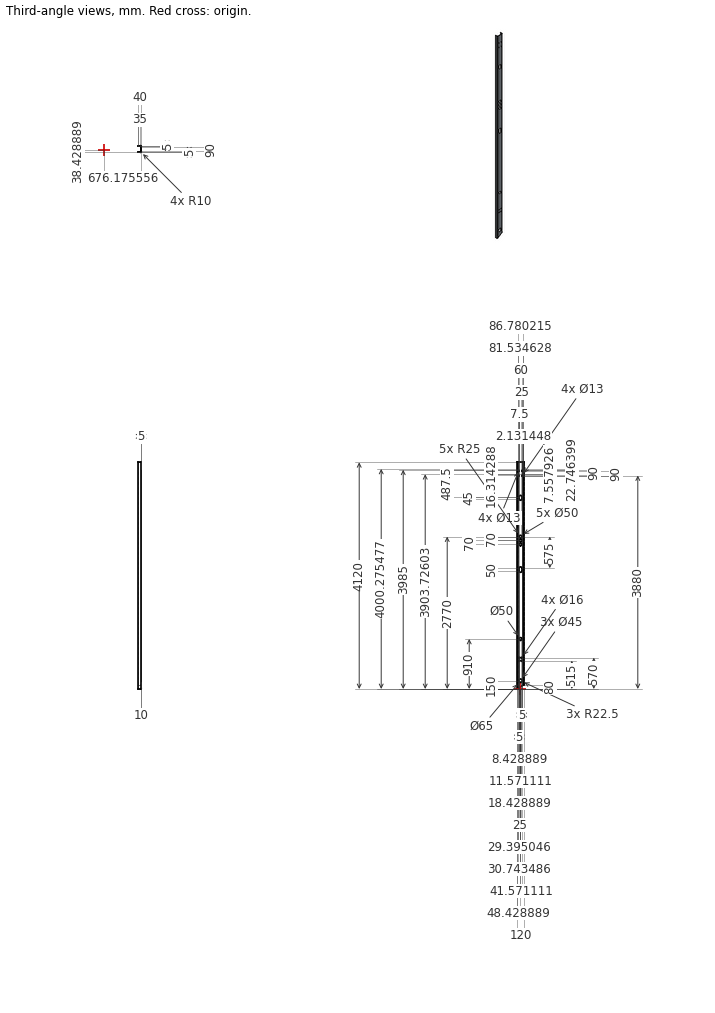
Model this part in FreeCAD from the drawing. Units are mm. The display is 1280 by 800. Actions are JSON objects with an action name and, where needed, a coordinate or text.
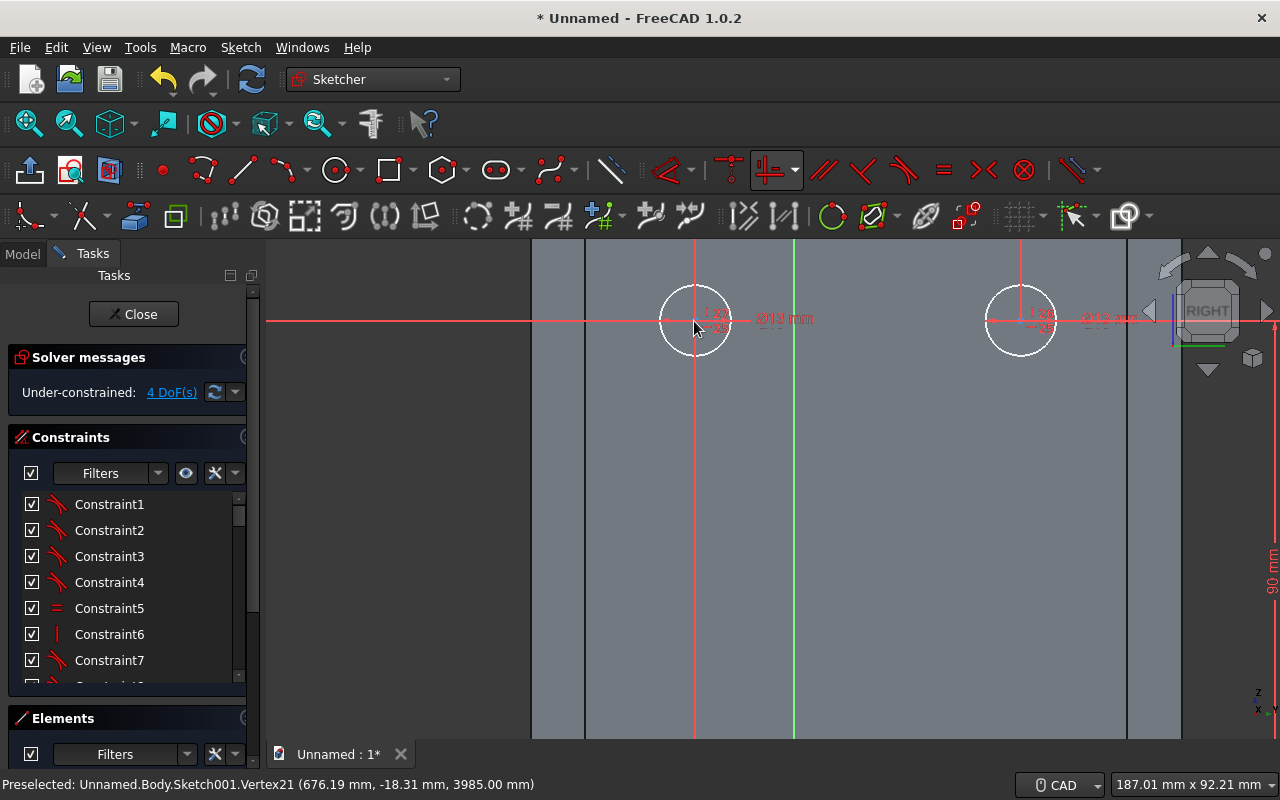
{"action": "scroll", "coordinate": [704, 489], "scroll_direction": "down", "scroll_amount": 15}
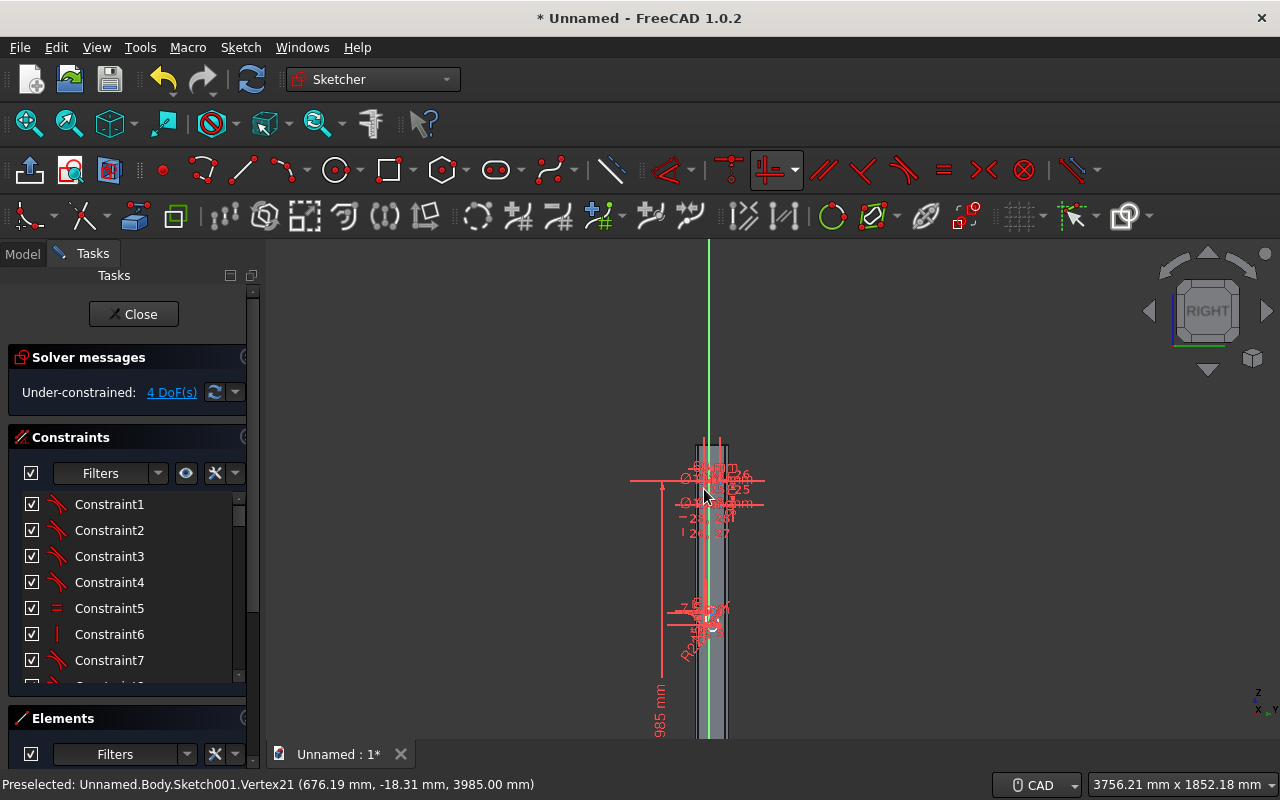
{"action": "scroll", "coordinate": [701, 267], "scroll_direction": "down", "scroll_amount": 6}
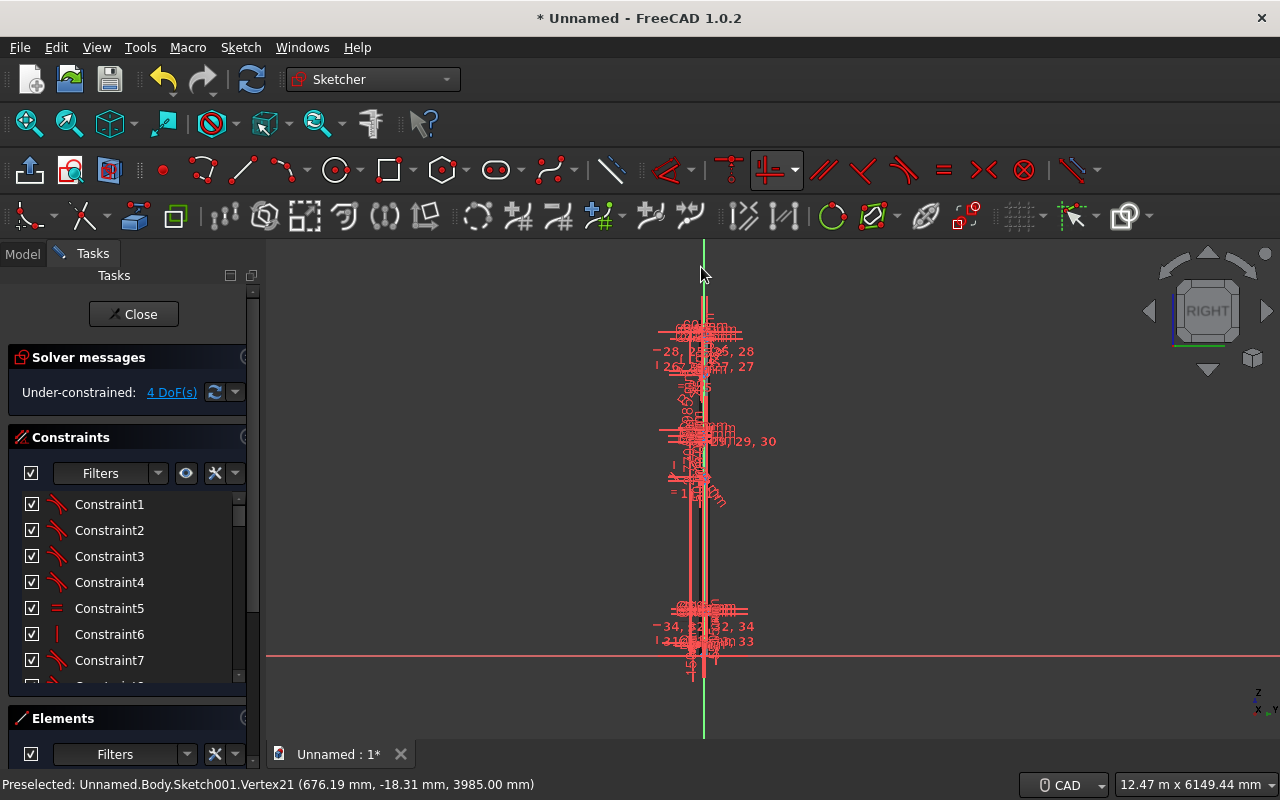
{"action": "scroll", "coordinate": [707, 477], "scroll_direction": "up", "scroll_amount": 9}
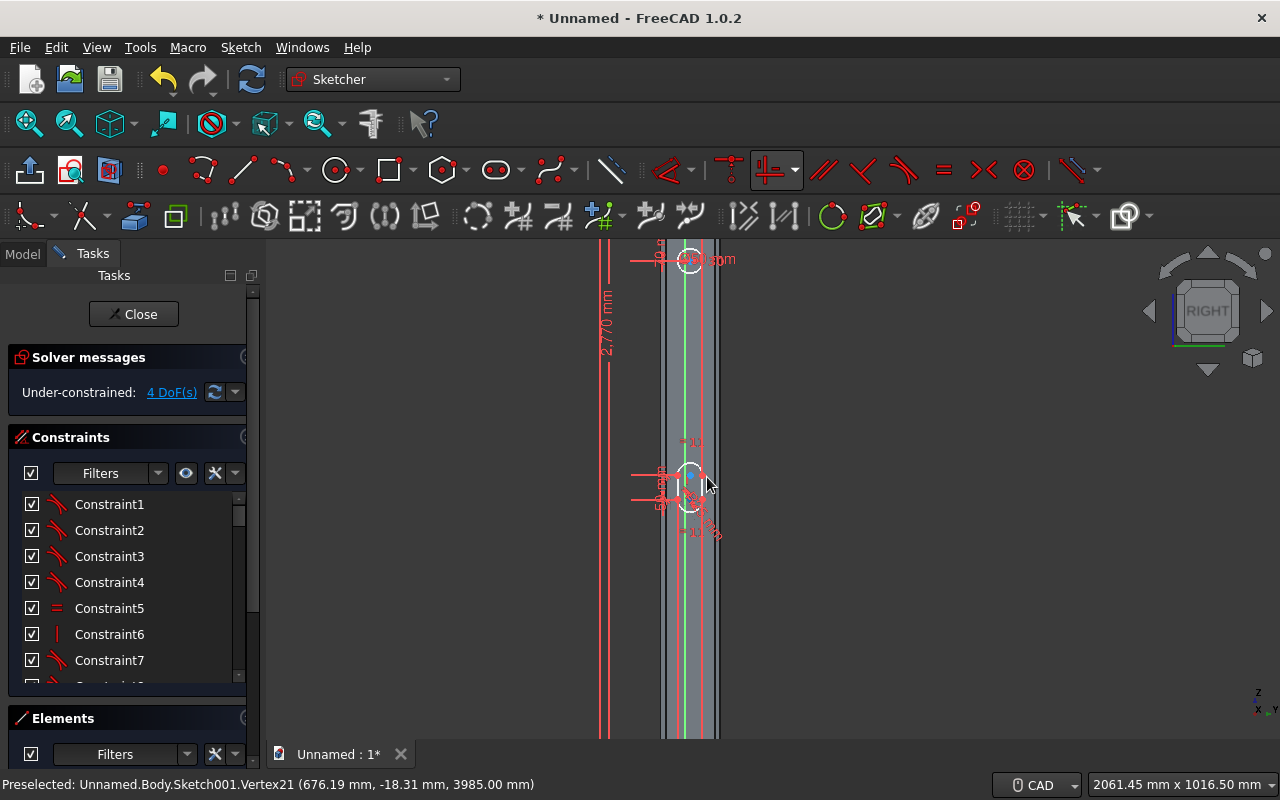
{"action": "left_click", "coordinate": [702, 475]}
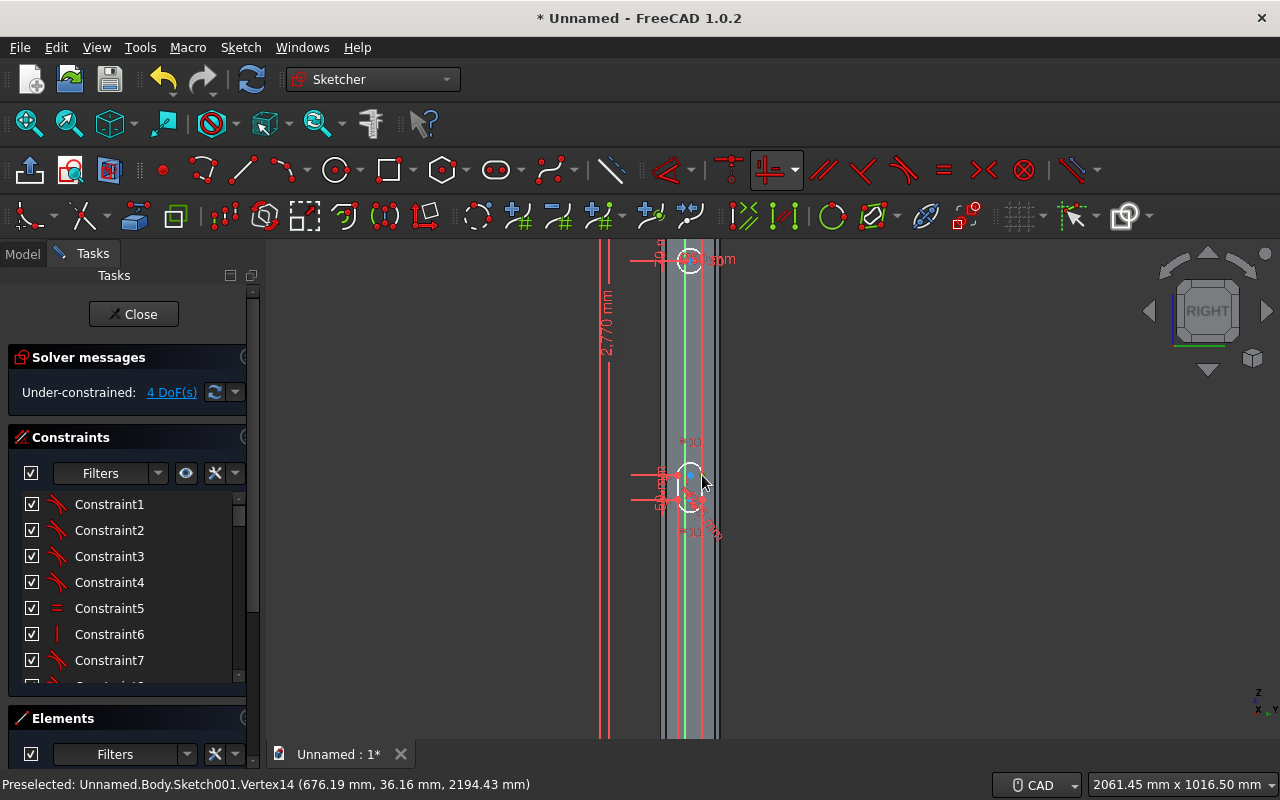
{"action": "scroll", "coordinate": [707, 472], "scroll_direction": "down", "scroll_amount": 9}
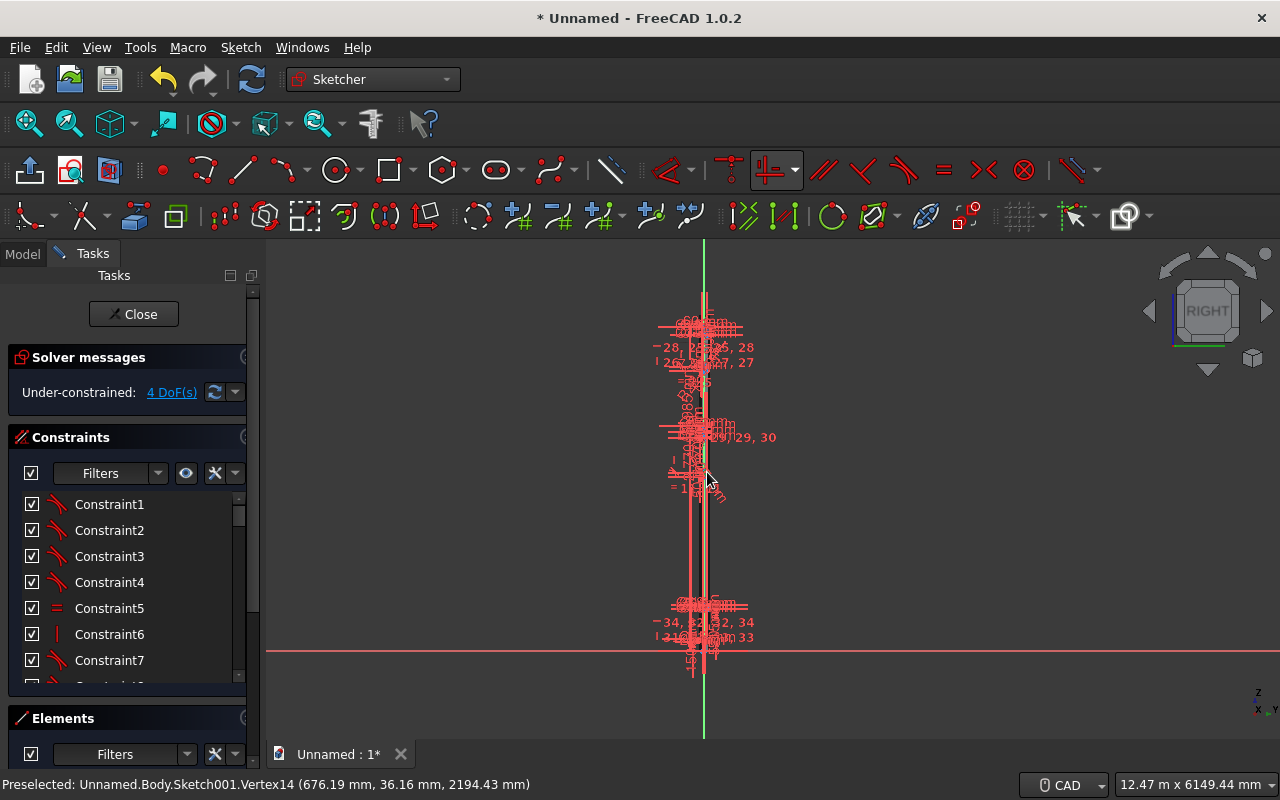
{"action": "scroll", "coordinate": [705, 426], "scroll_direction": "up", "scroll_amount": 4}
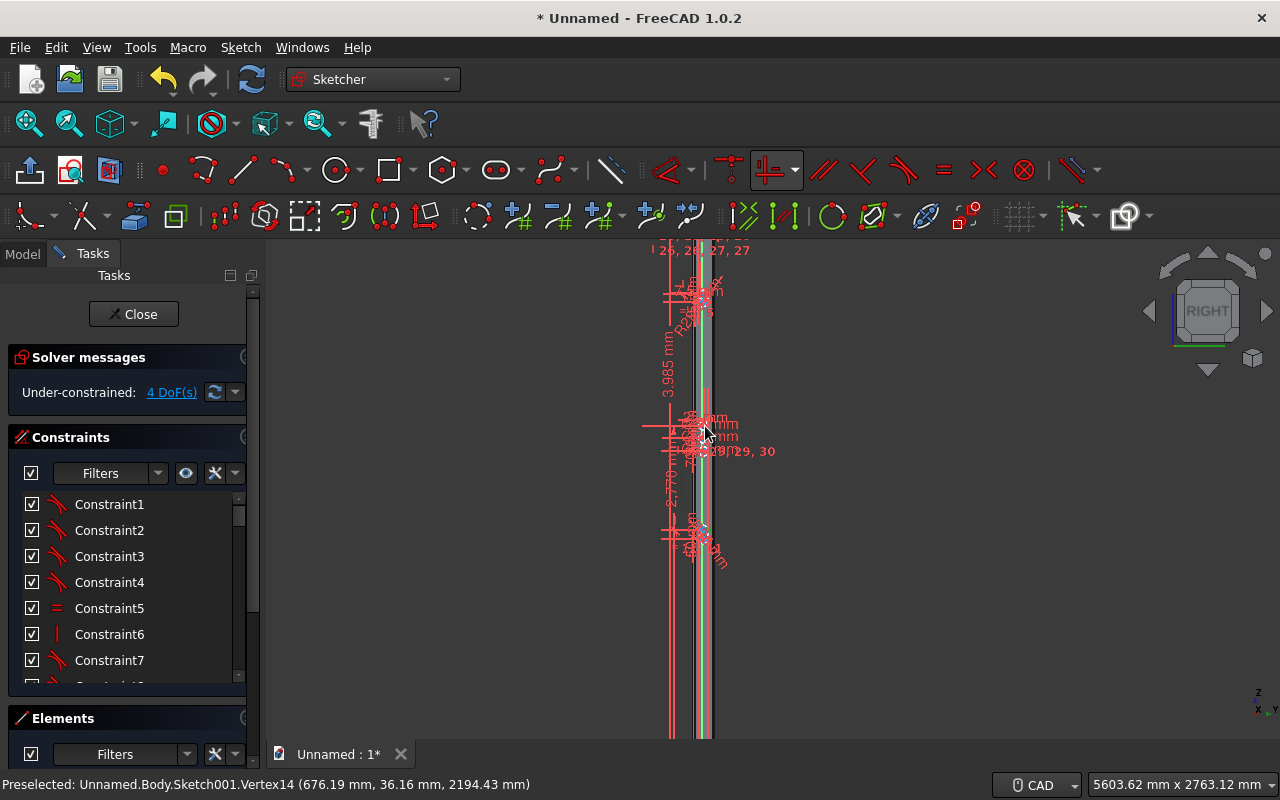
{"action": "left_click", "coordinate": [704, 426]}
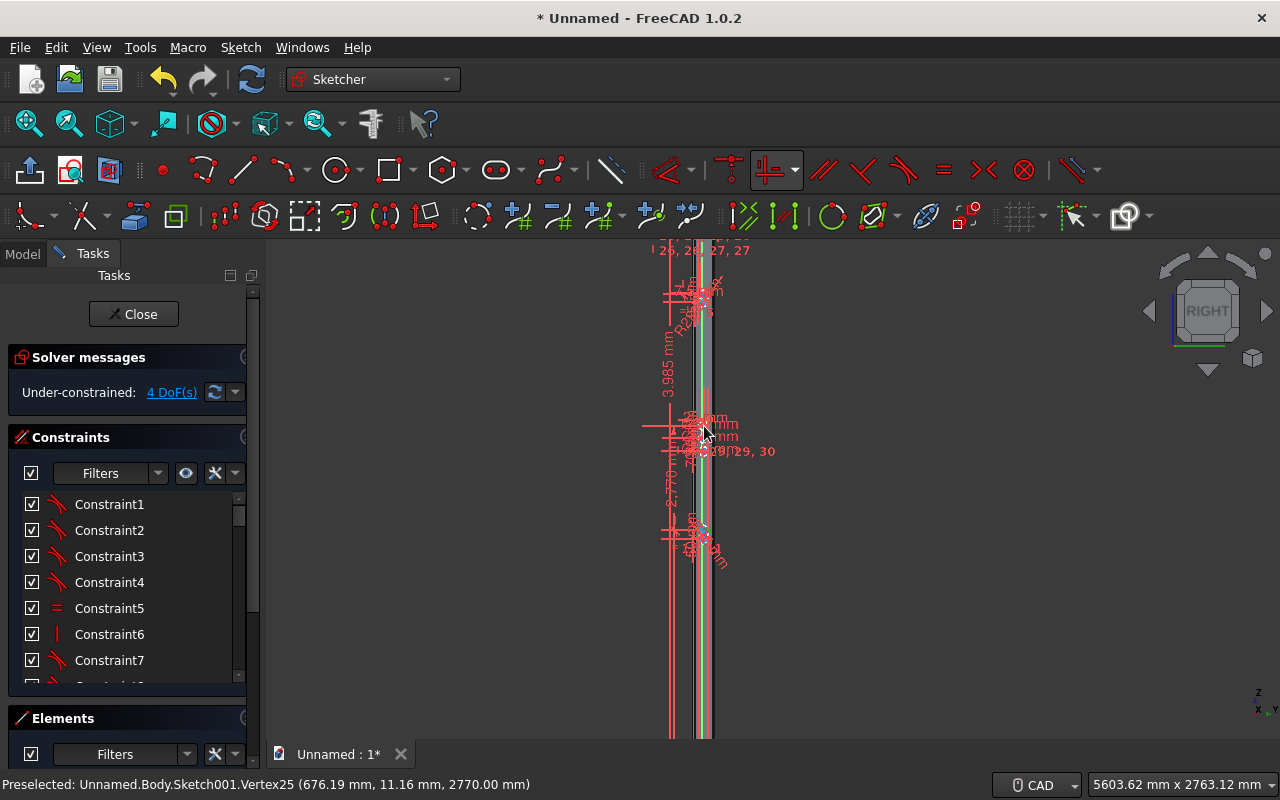
{"action": "left_click", "coordinate": [694, 170]}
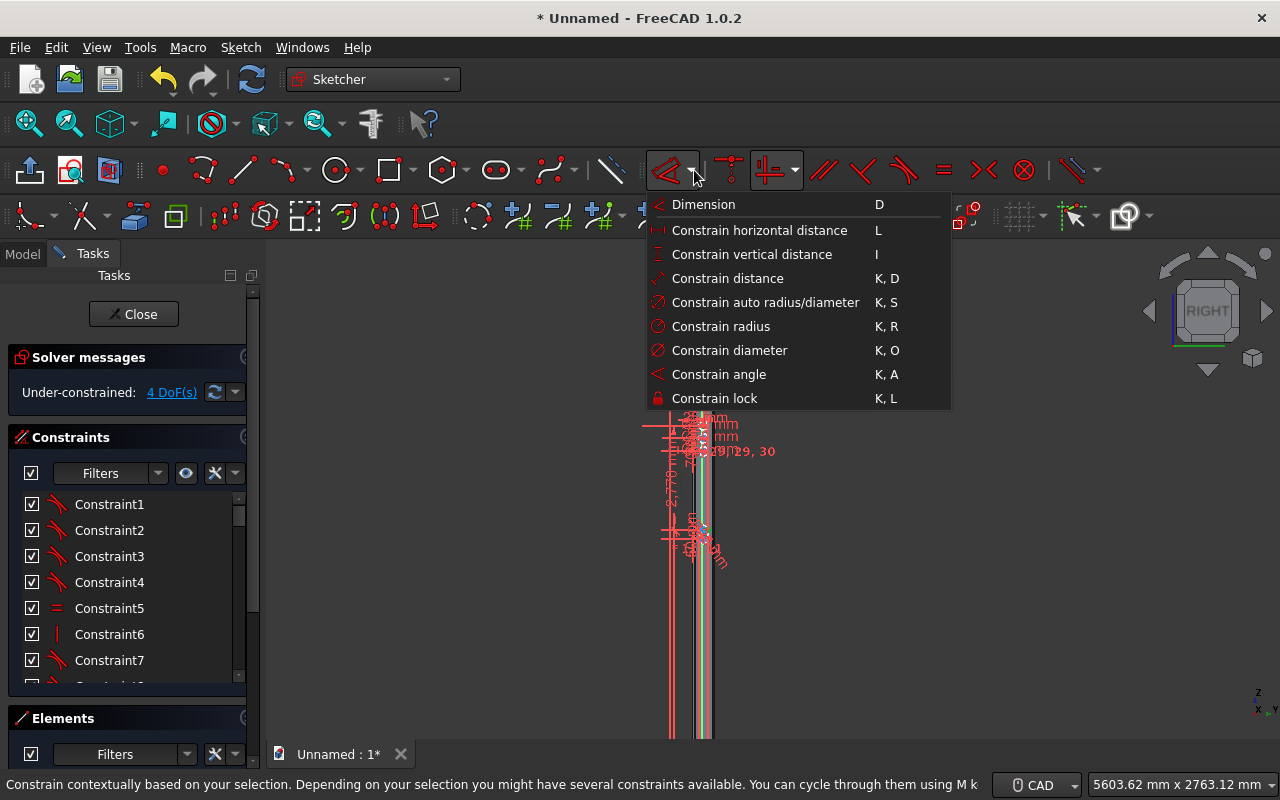
{"action": "left_click", "coordinate": [799, 254]}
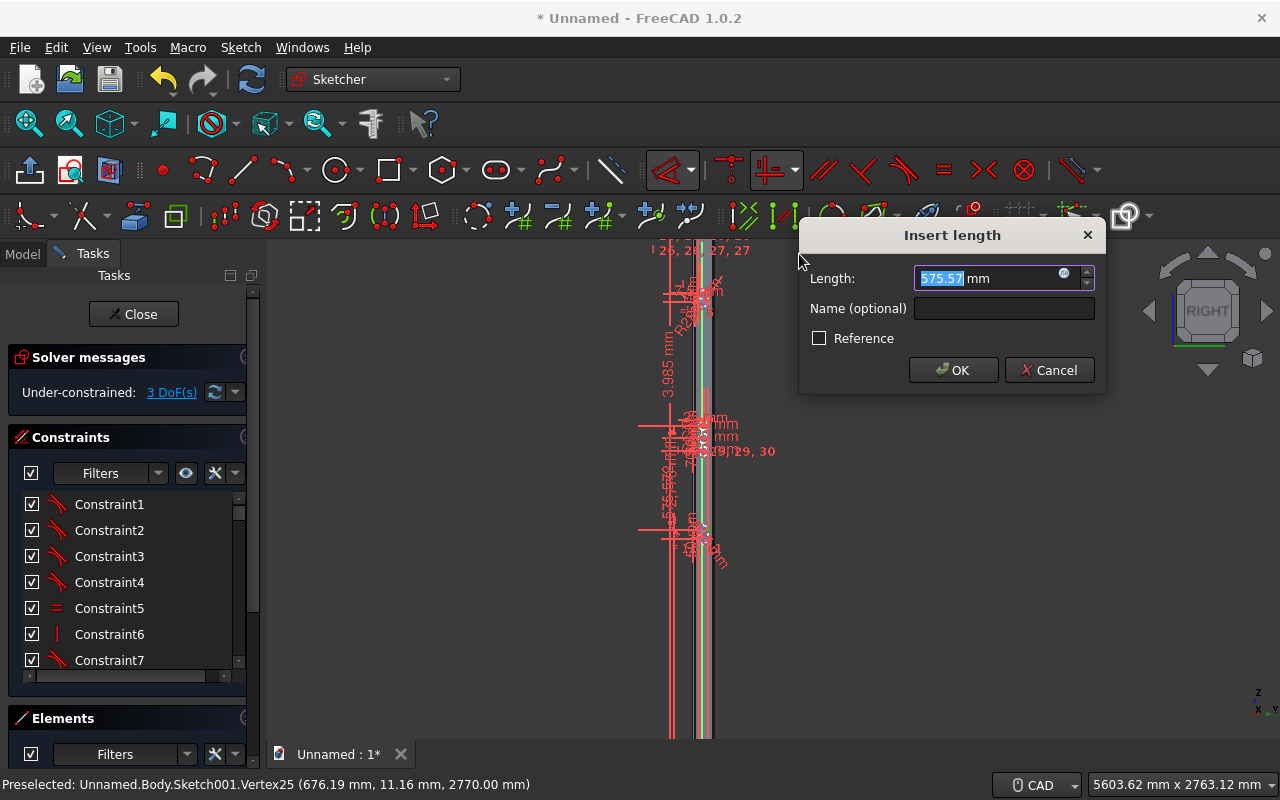
{"action": "type", "text": "575"}
{"action": "key", "text": "Return"}